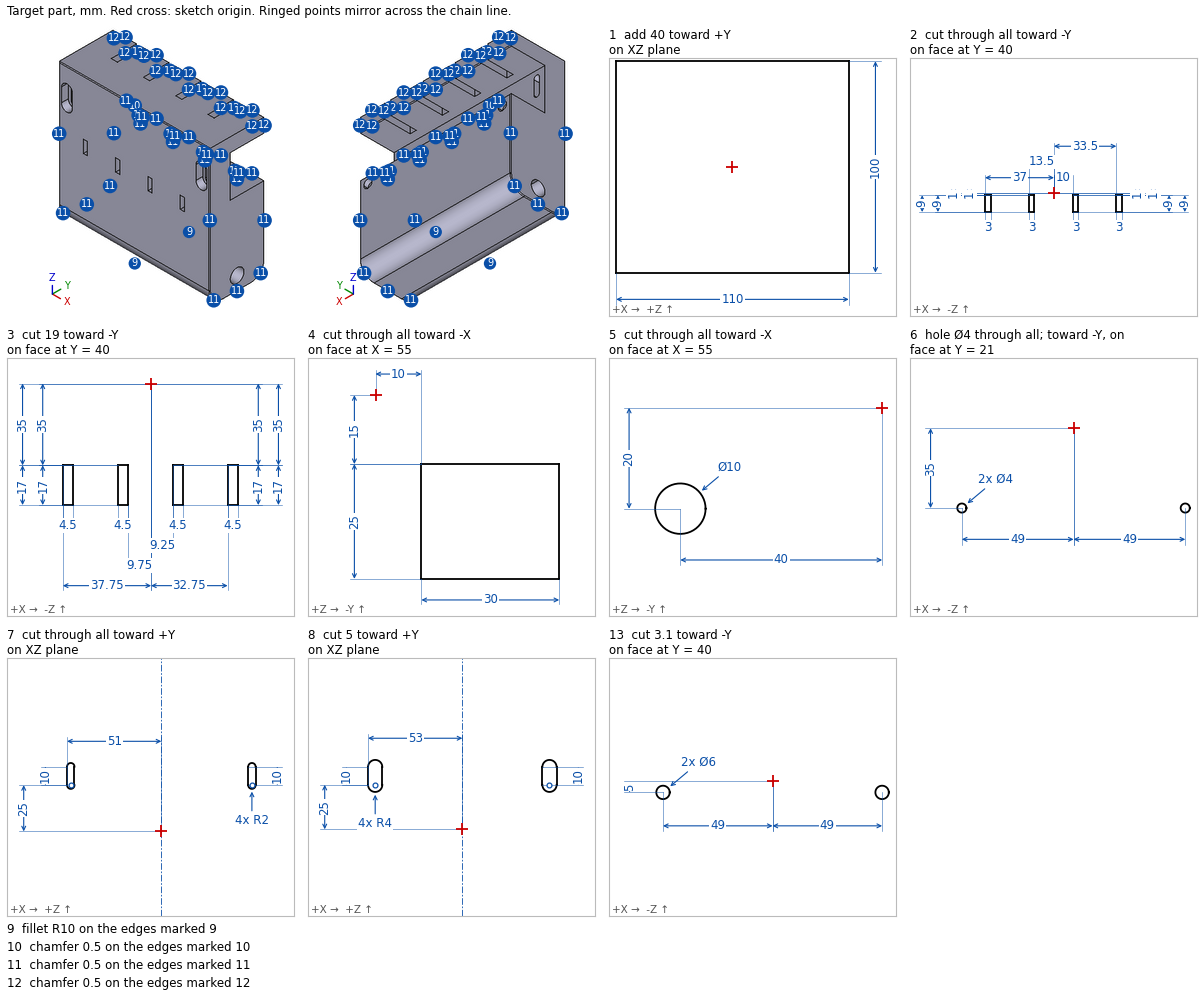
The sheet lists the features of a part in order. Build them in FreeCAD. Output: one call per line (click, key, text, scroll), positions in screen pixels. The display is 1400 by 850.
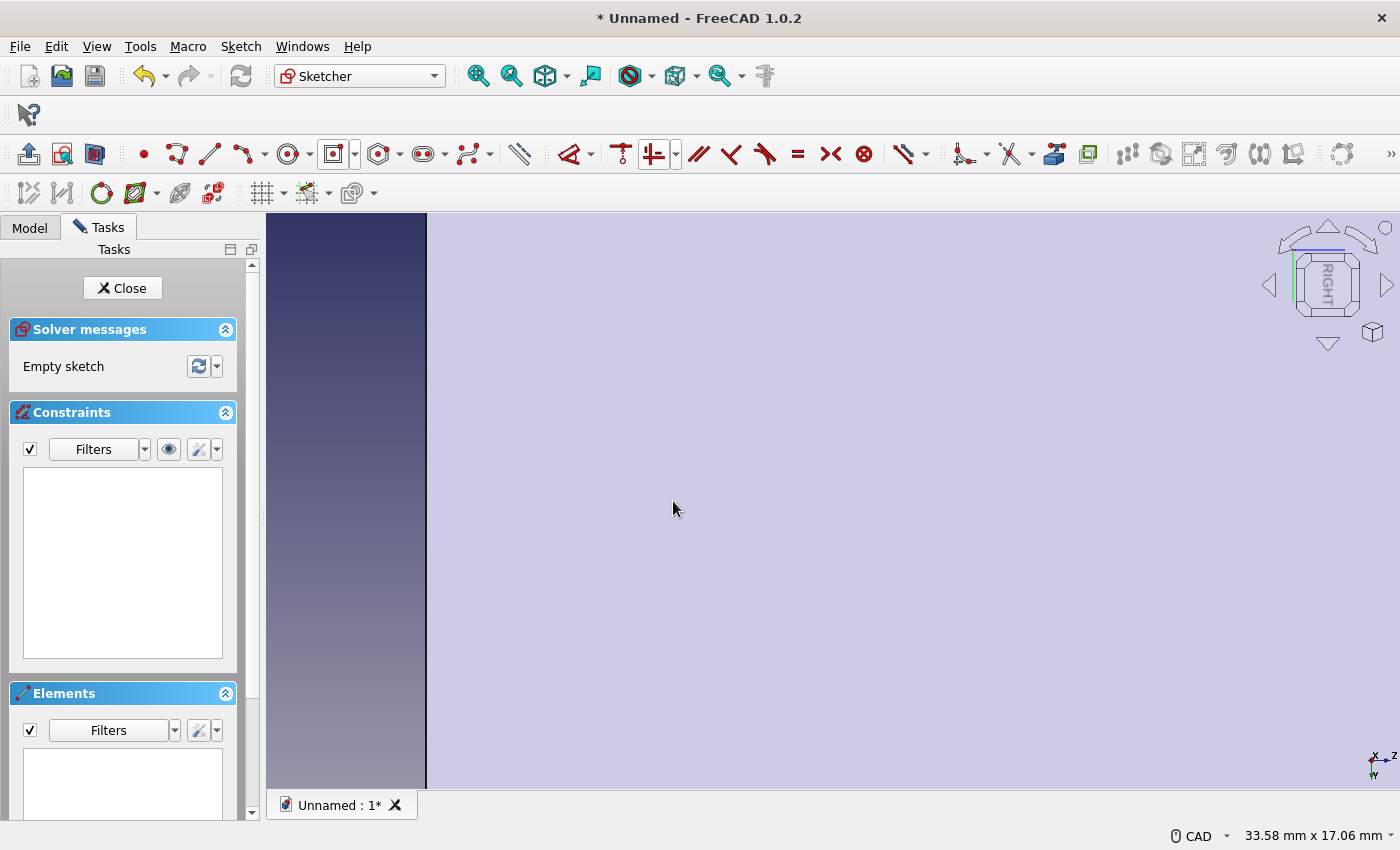
click(288, 154)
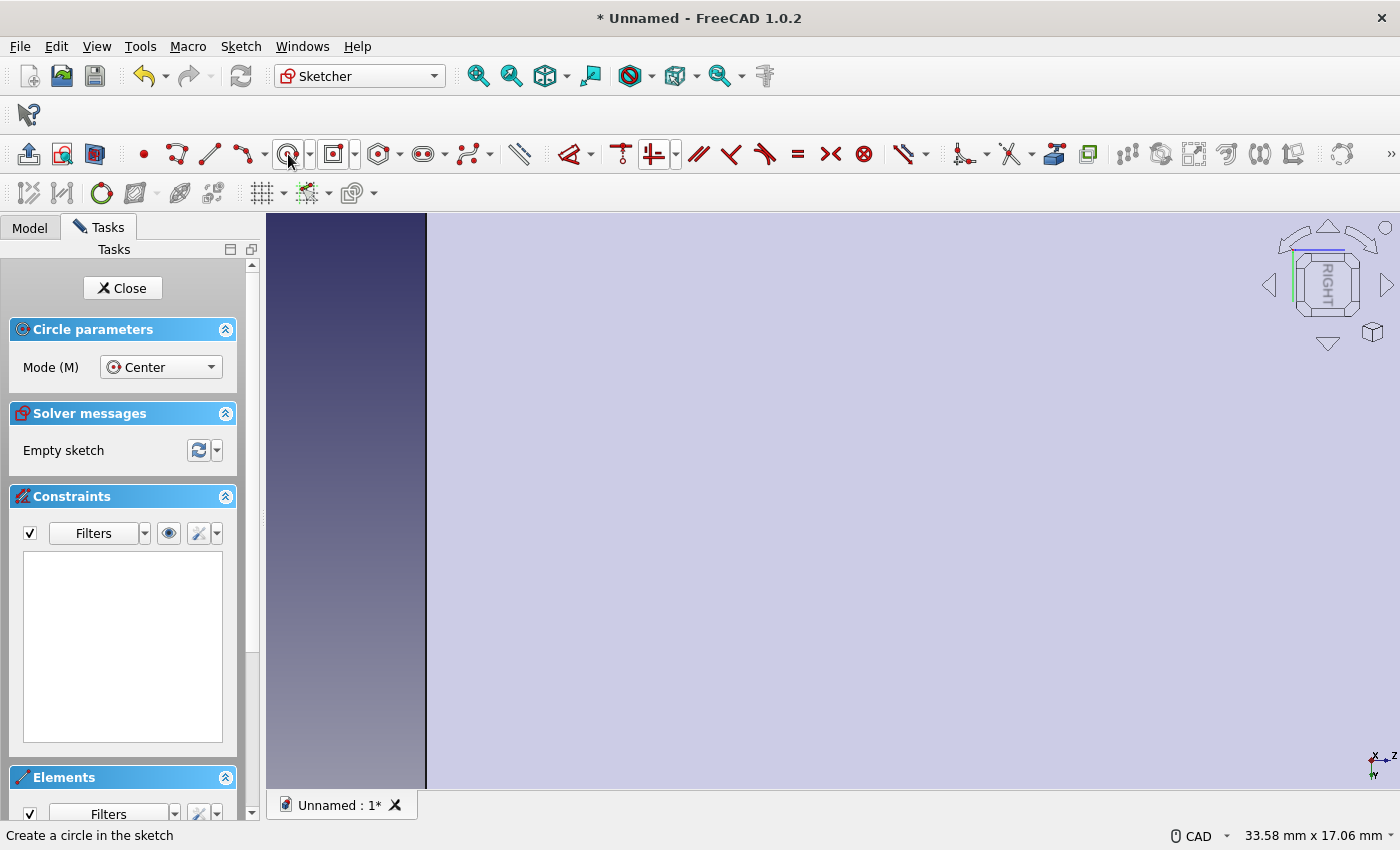
click(763, 497)
click(883, 378)
key(Escape)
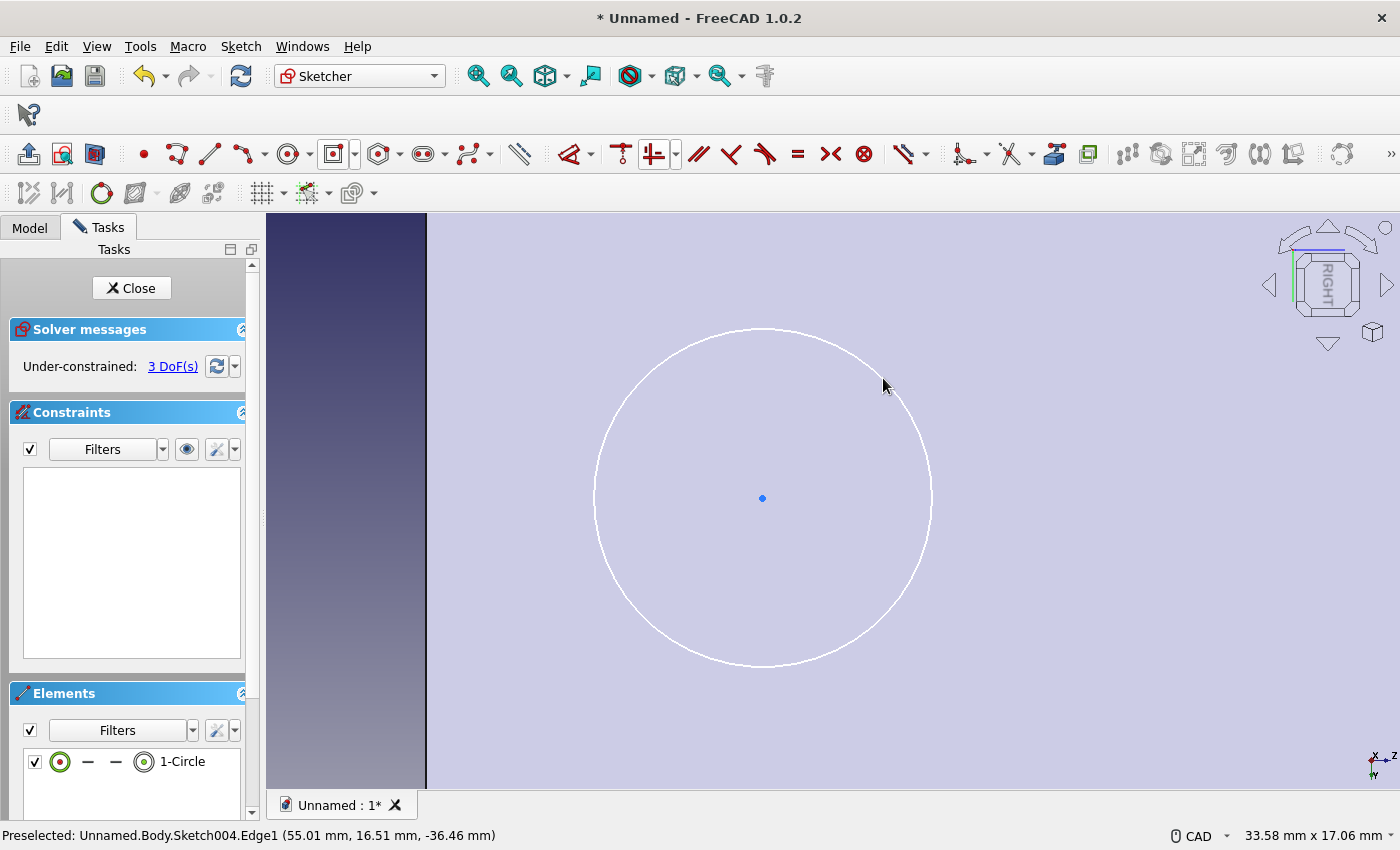
key(d)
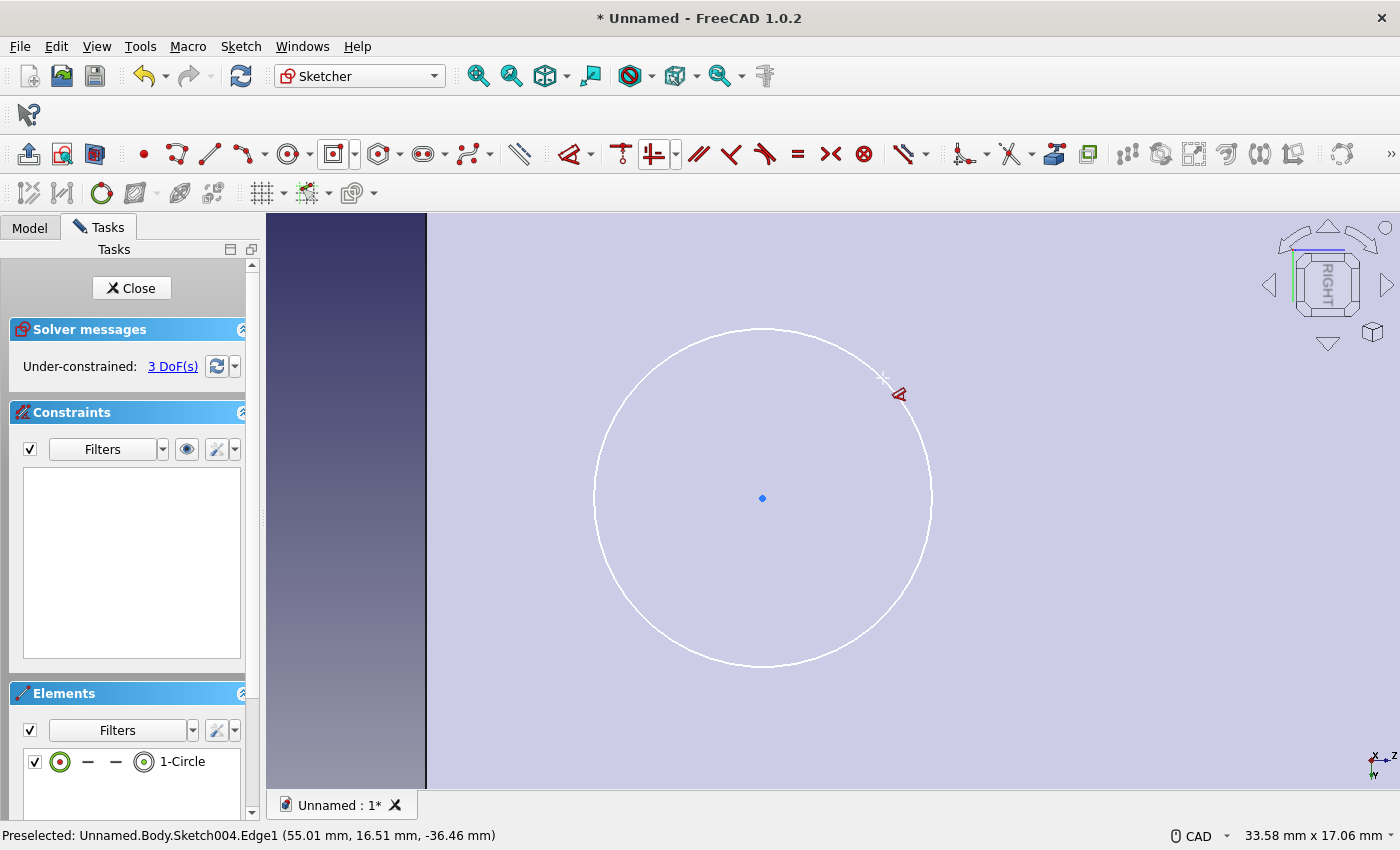
click(882, 378)
click(905, 355)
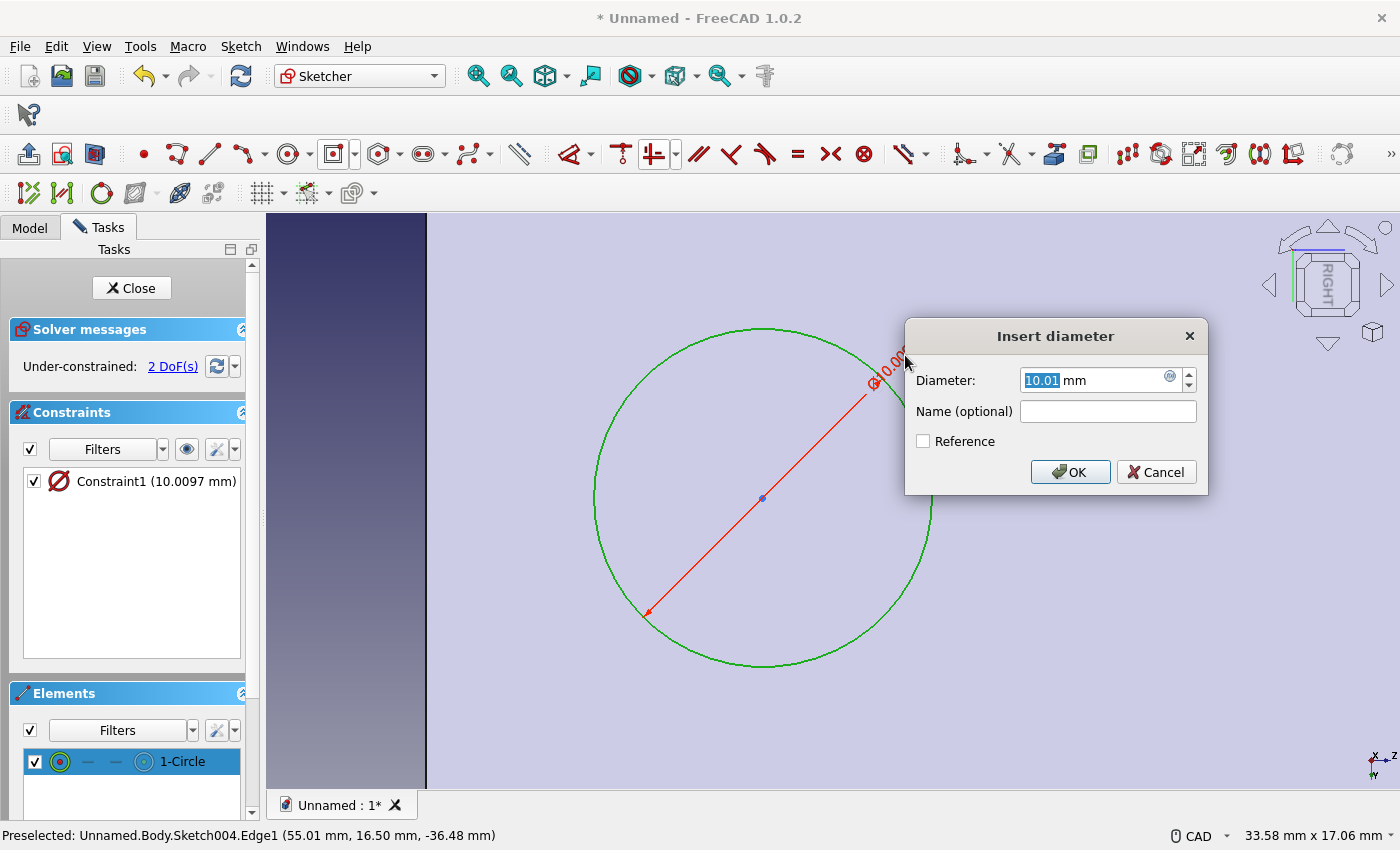
text(10)
key(Return)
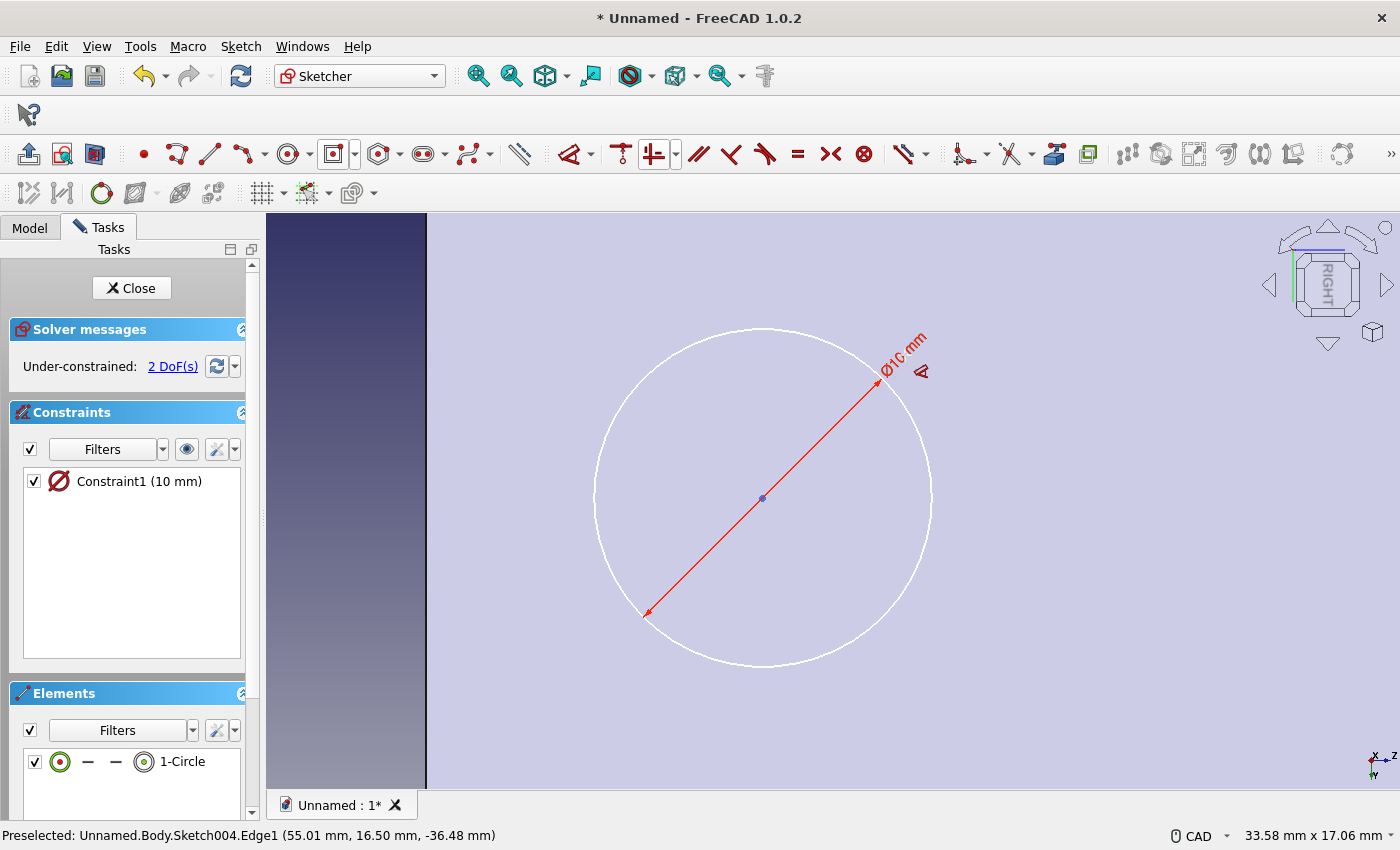
click(763, 498)
click(999, 532)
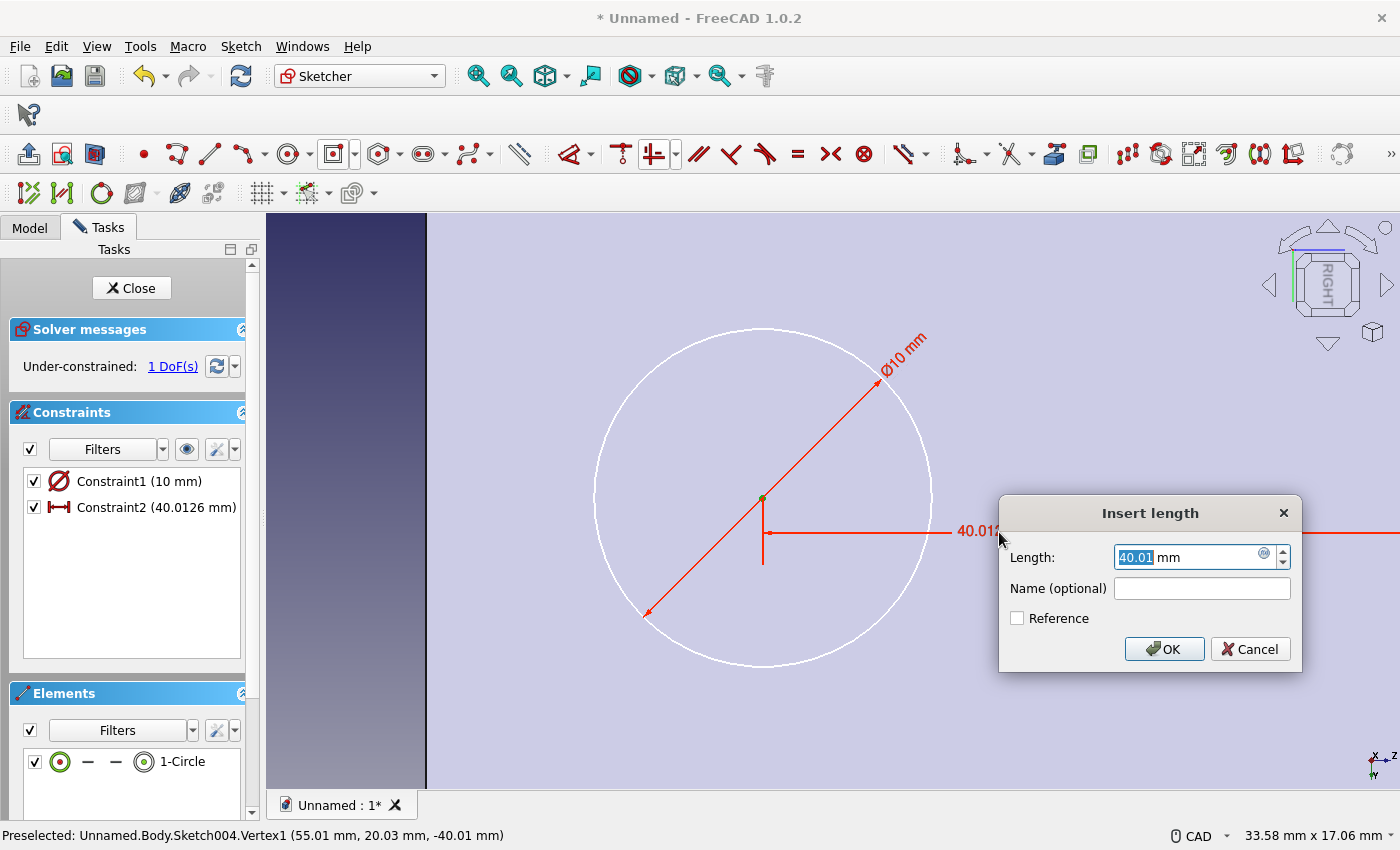
text(40)
key(Return)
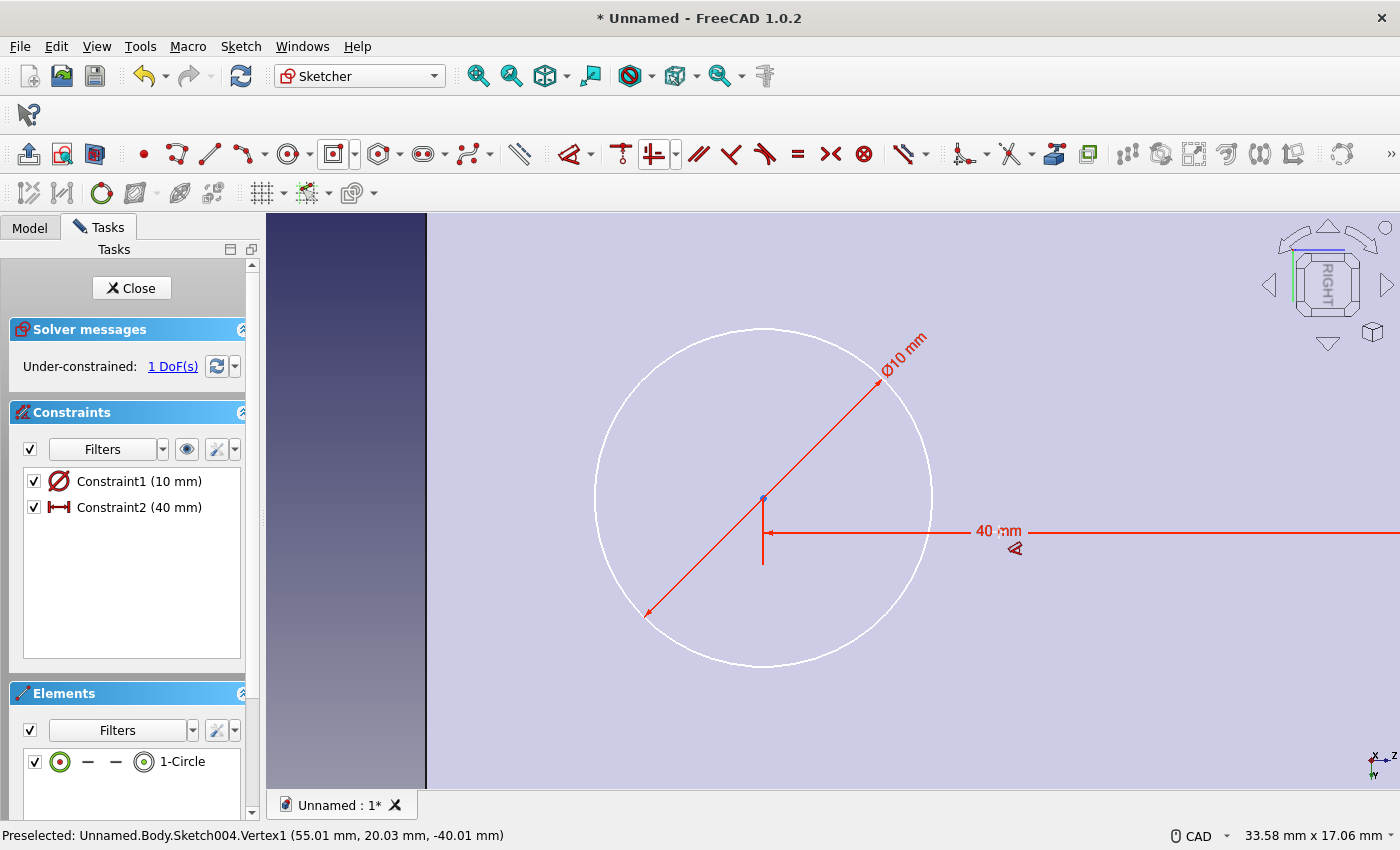
click(763, 498)
click(729, 370)